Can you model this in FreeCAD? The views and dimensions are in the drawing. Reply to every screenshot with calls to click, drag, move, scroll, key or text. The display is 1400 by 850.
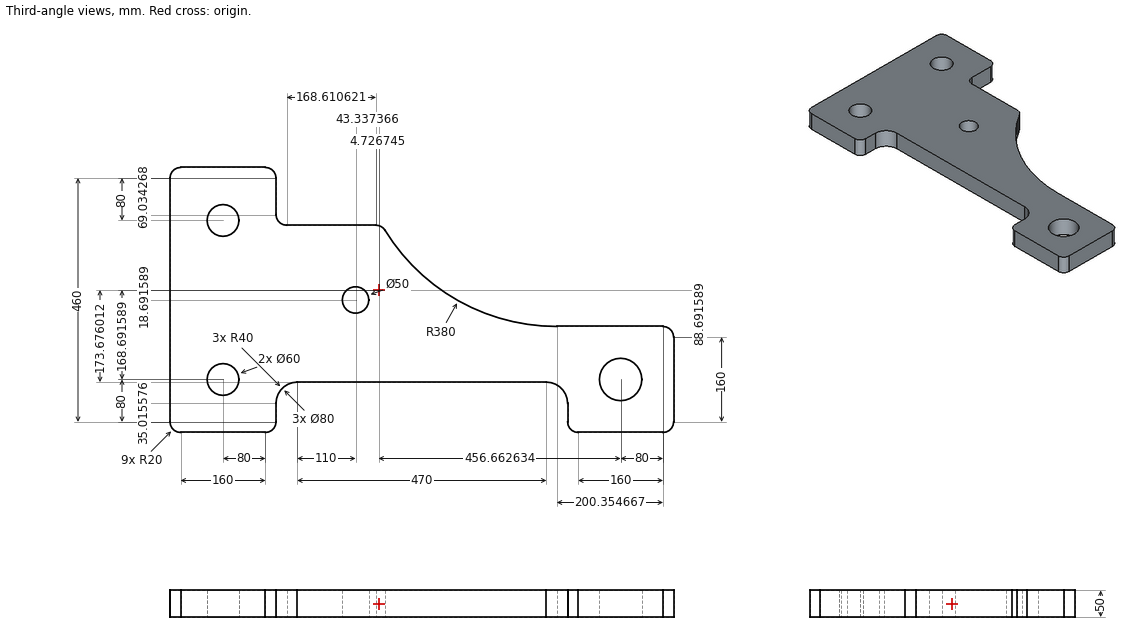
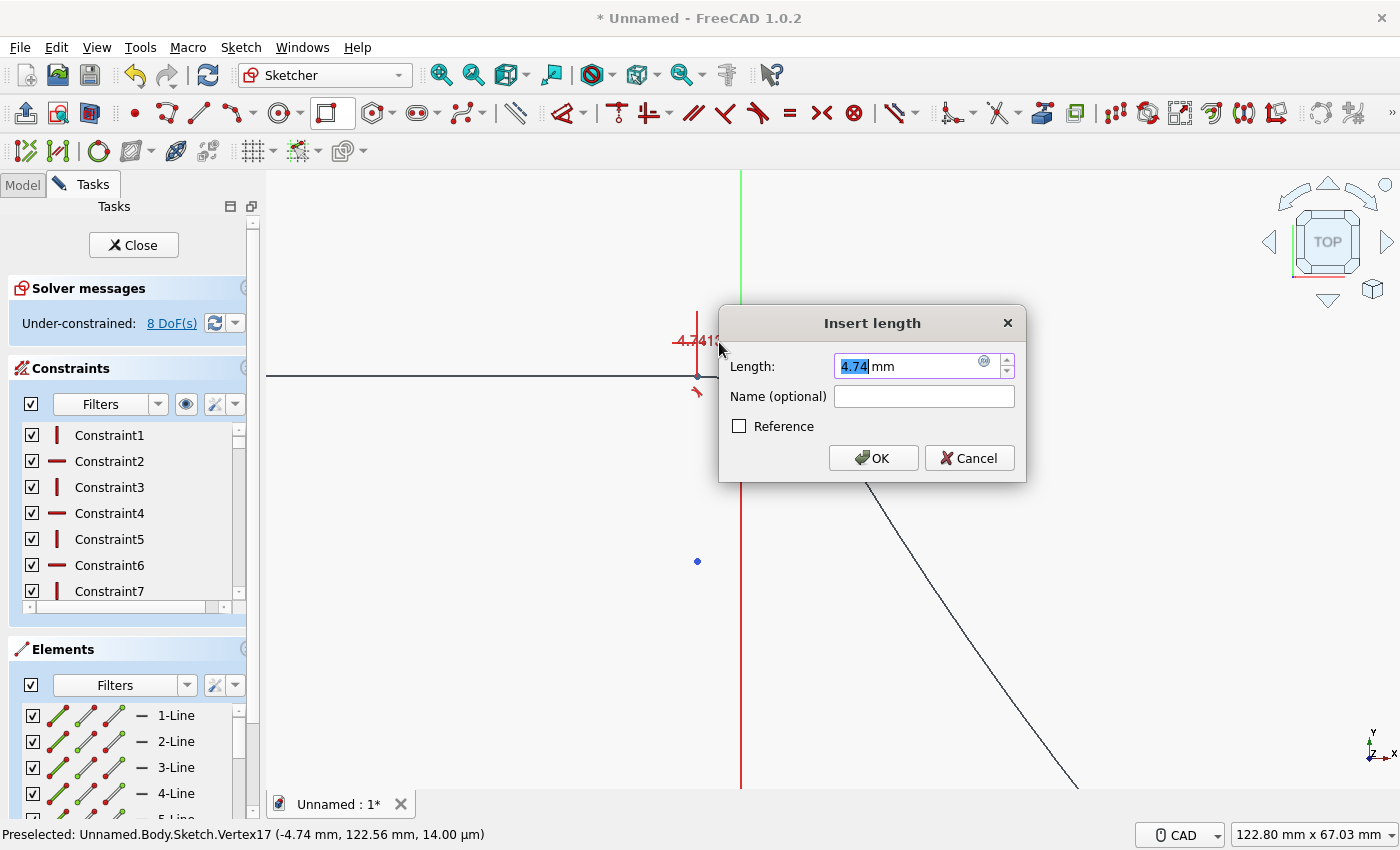
text(4.726745)
key(Return)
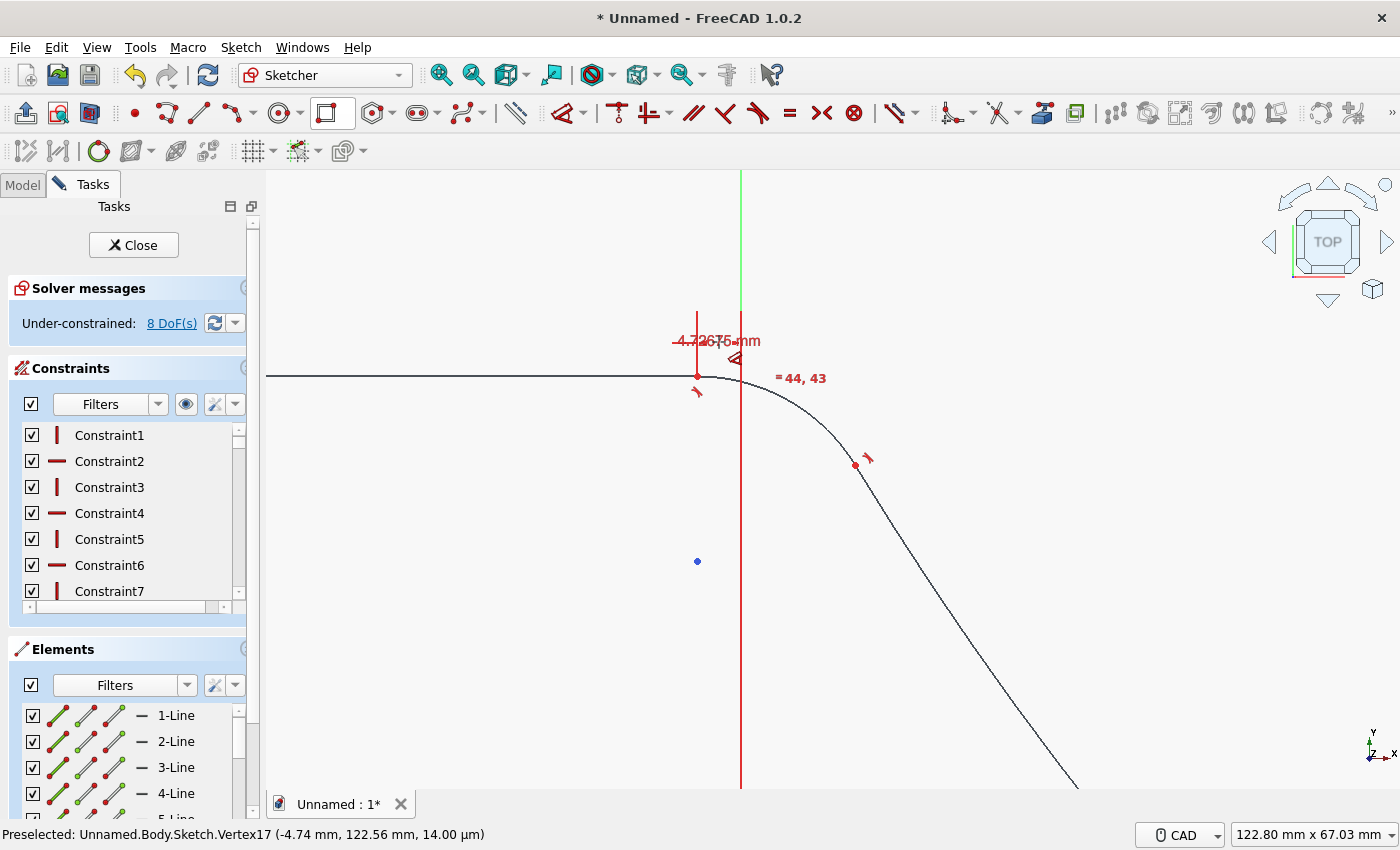
scroll(706, 383, down, 13)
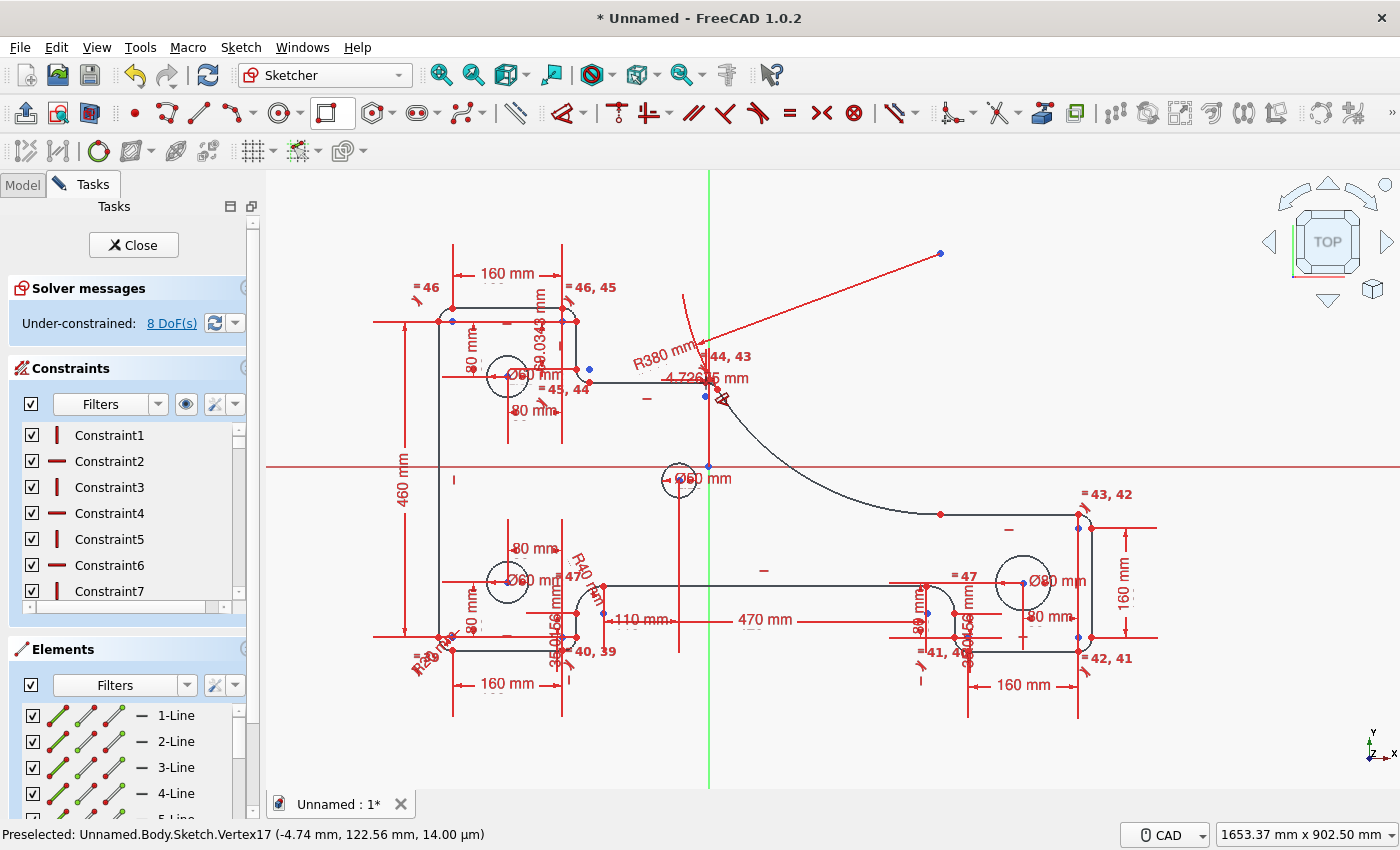
scroll(679, 481, up, 2)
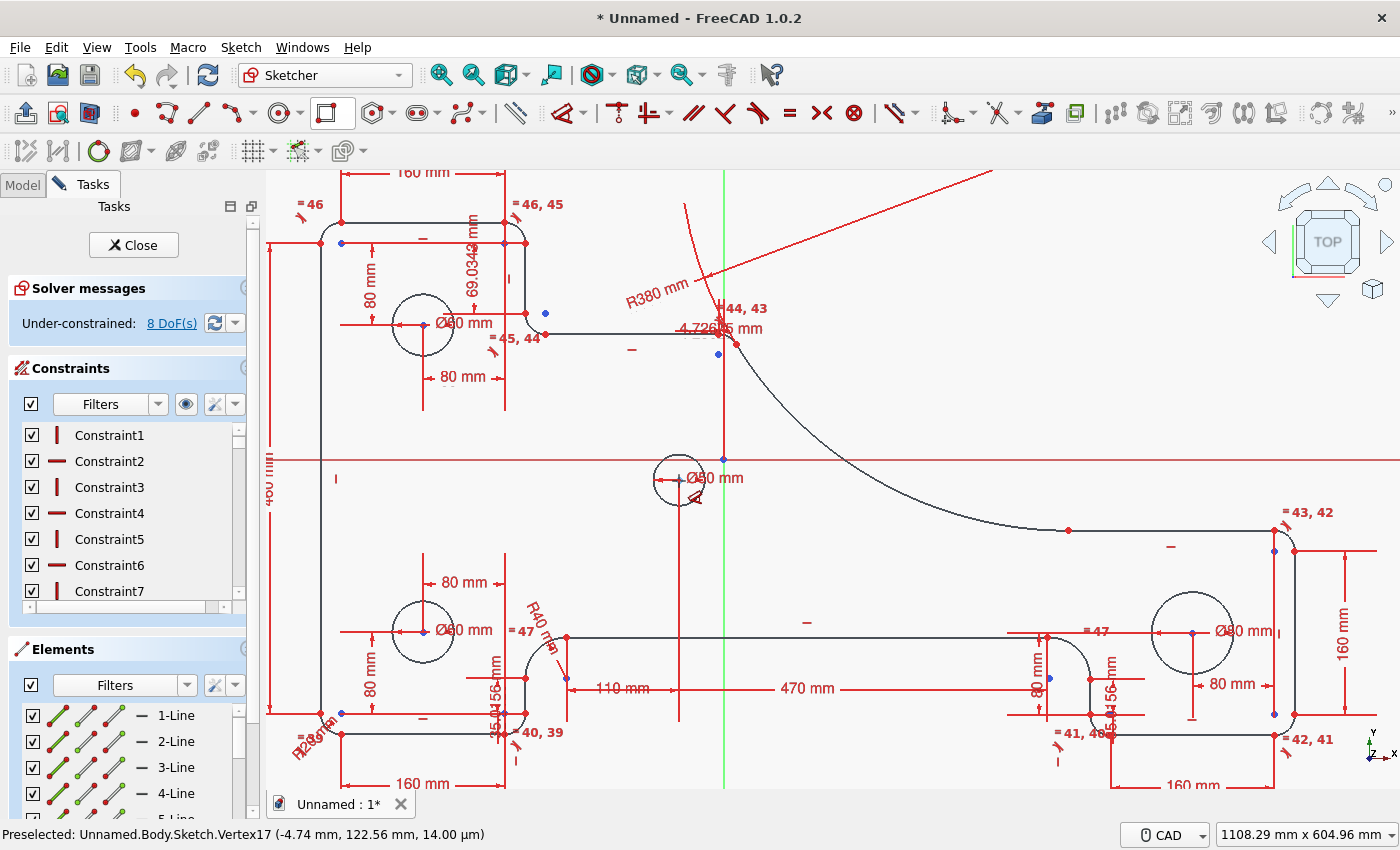
click(679, 480)
click(701, 426)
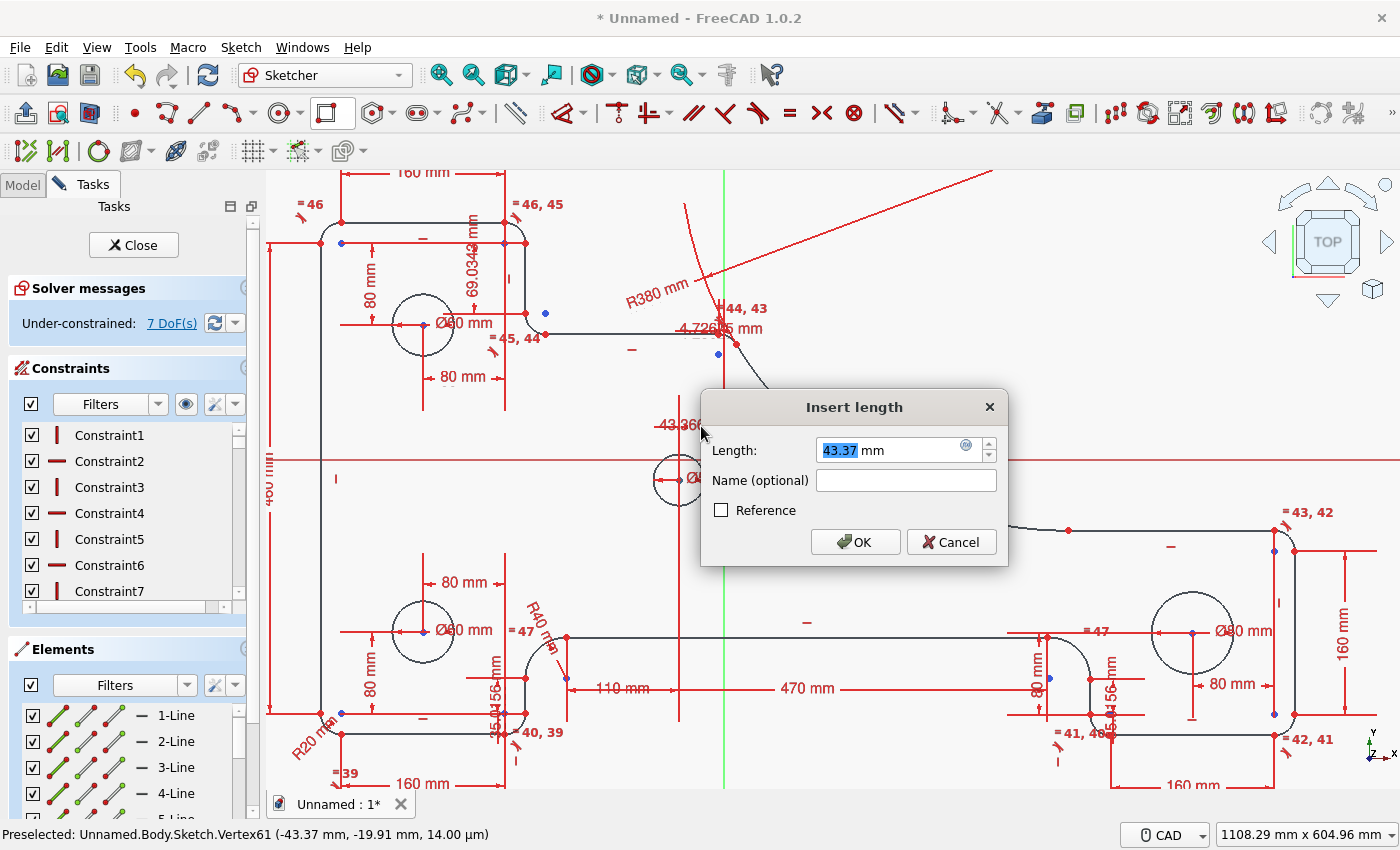
text(43.337366)
key(Return)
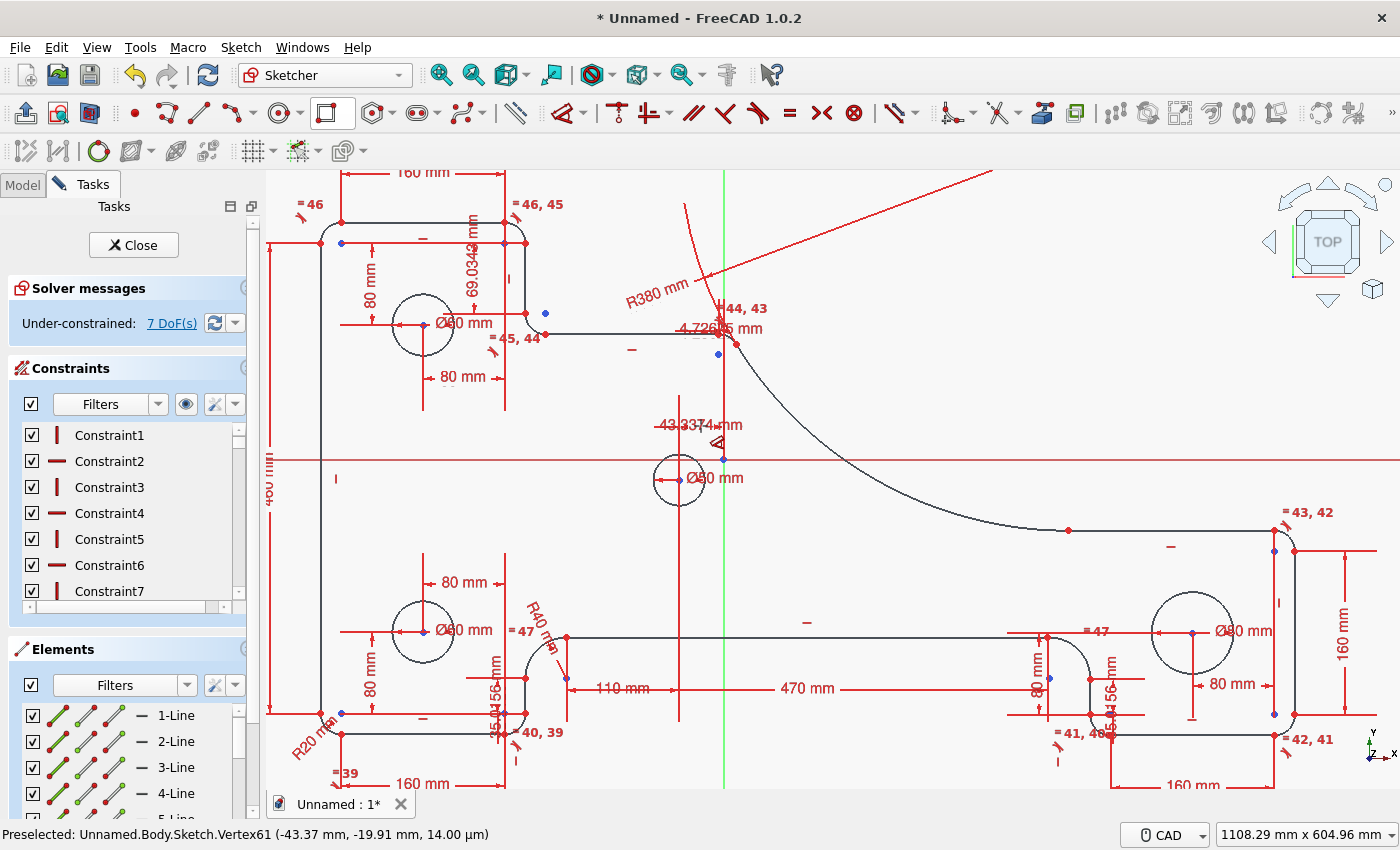
scroll(679, 480, up, 4)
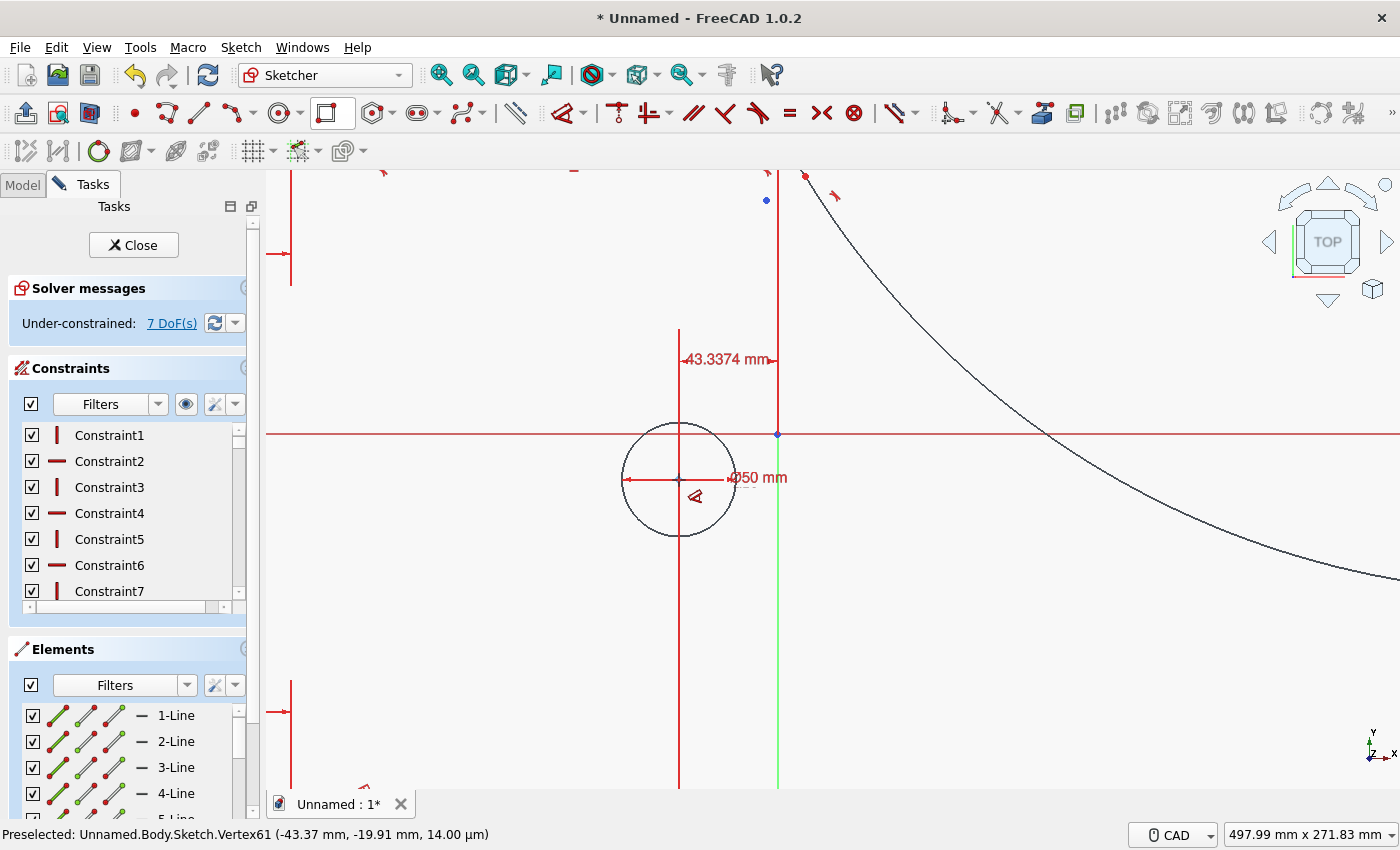
click(679, 480)
click(645, 457)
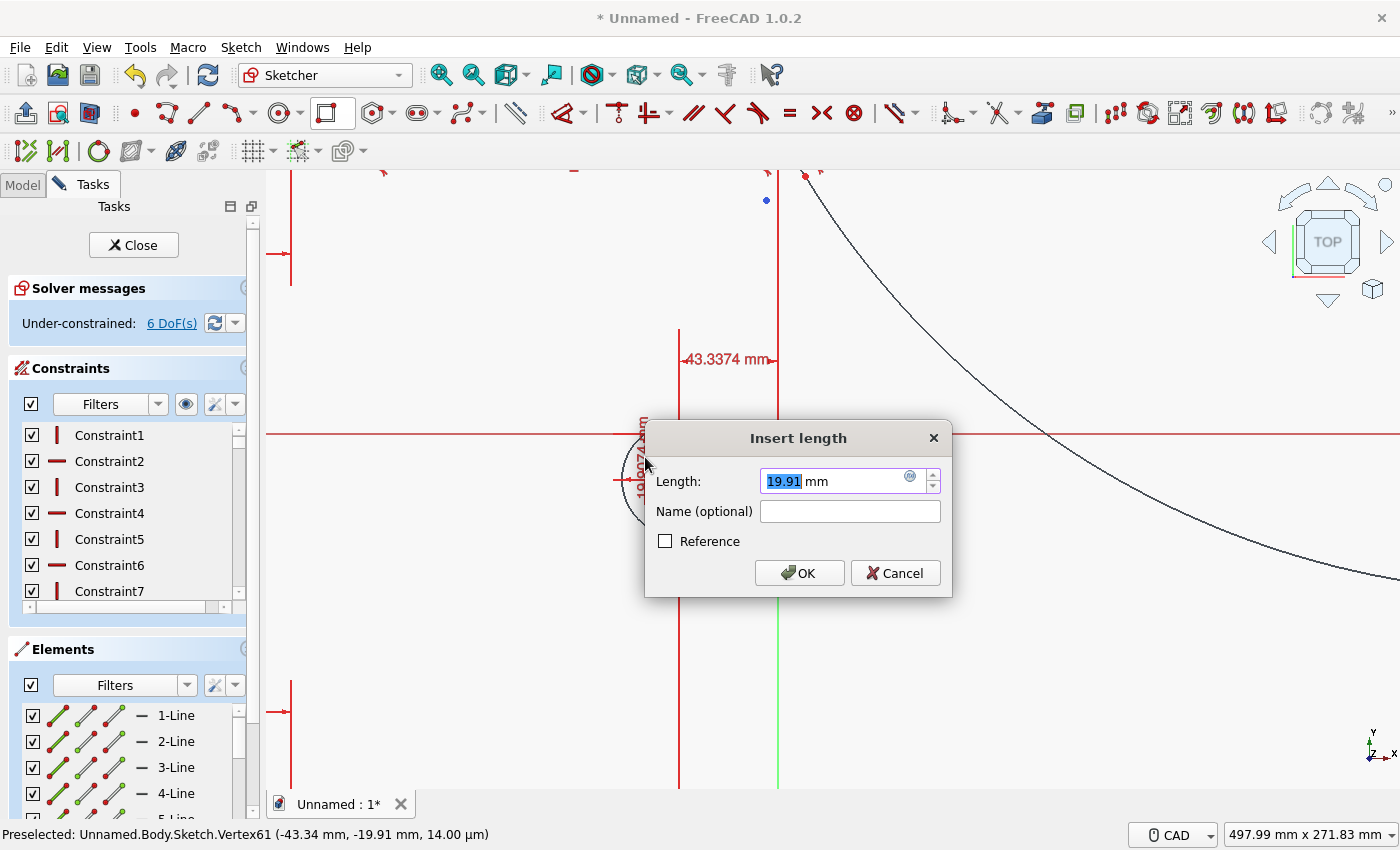
text(18.691589)
key(Return)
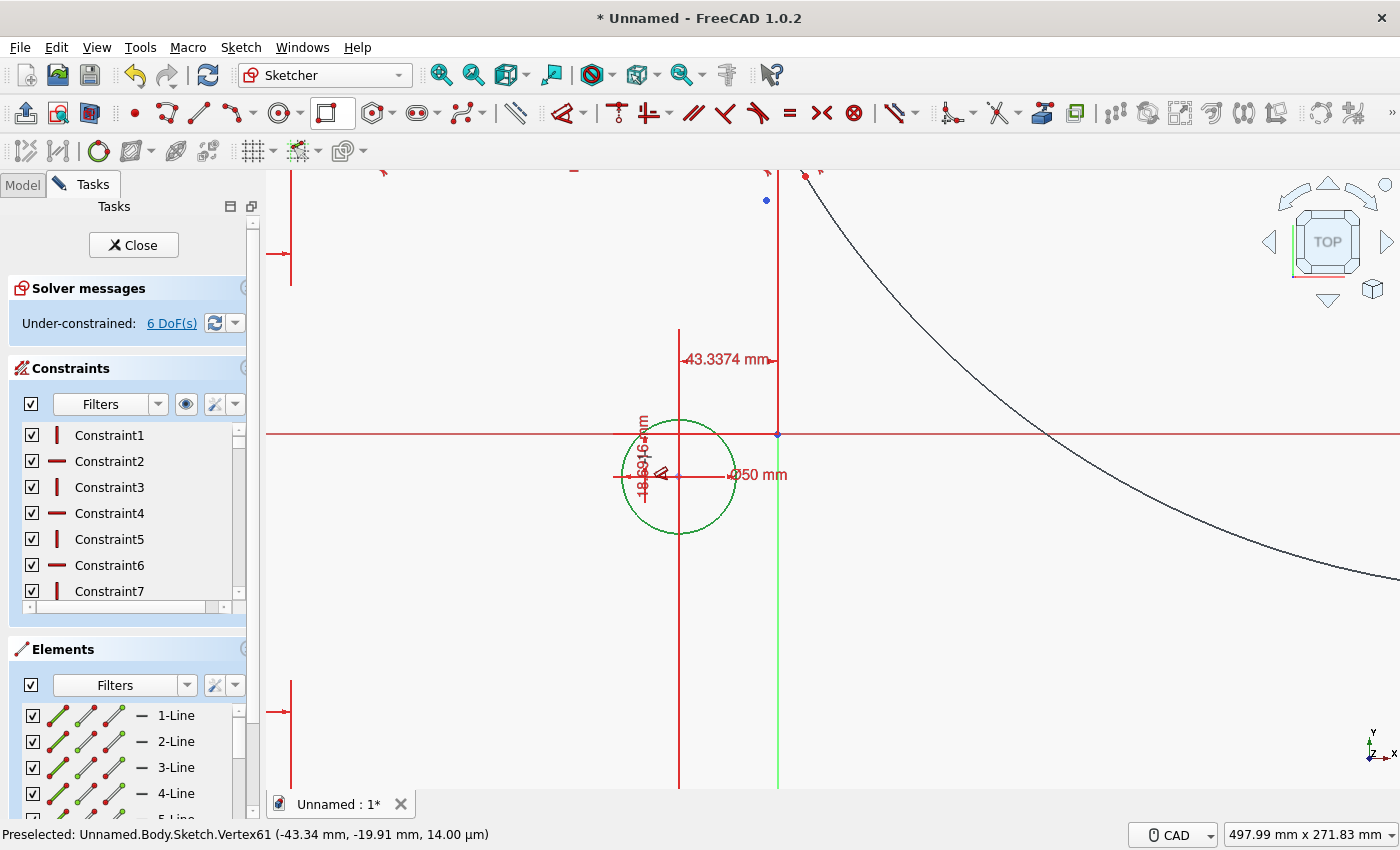
scroll(679, 481, down, 6)